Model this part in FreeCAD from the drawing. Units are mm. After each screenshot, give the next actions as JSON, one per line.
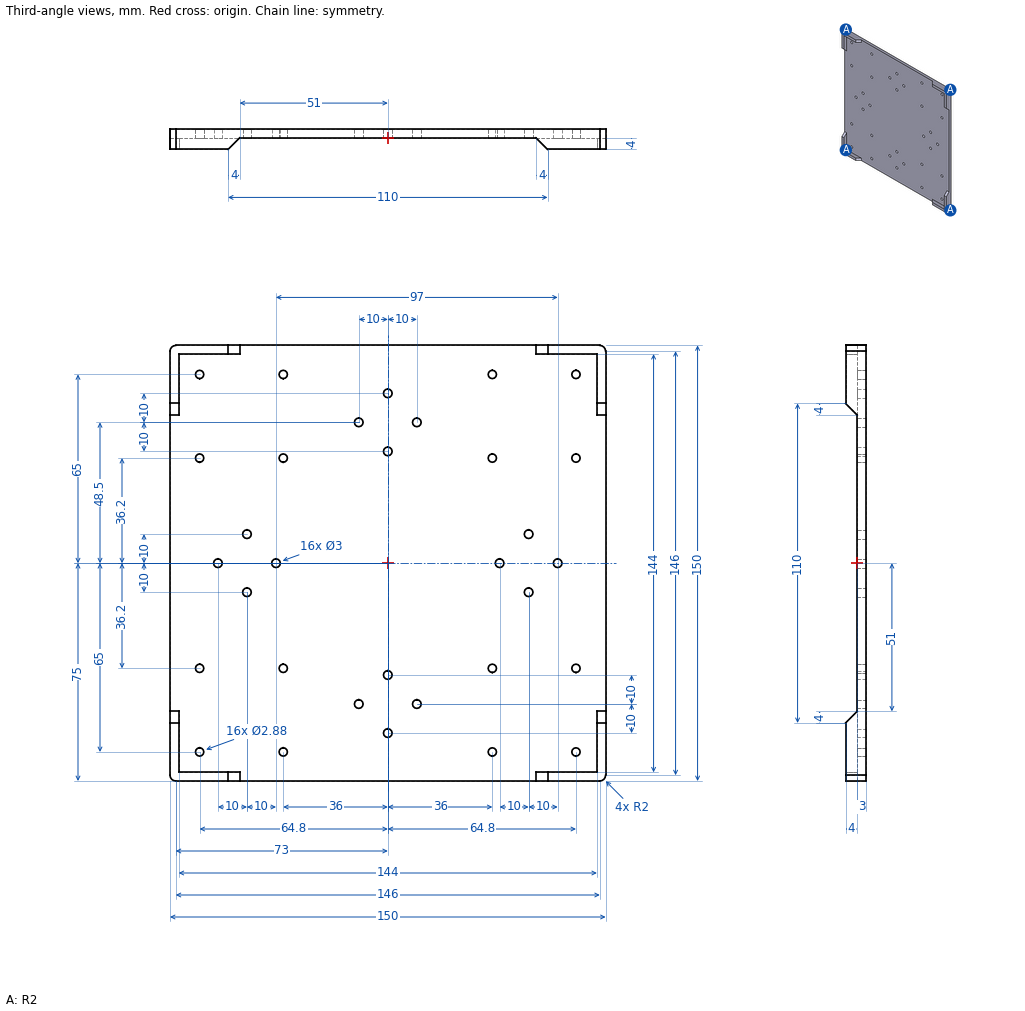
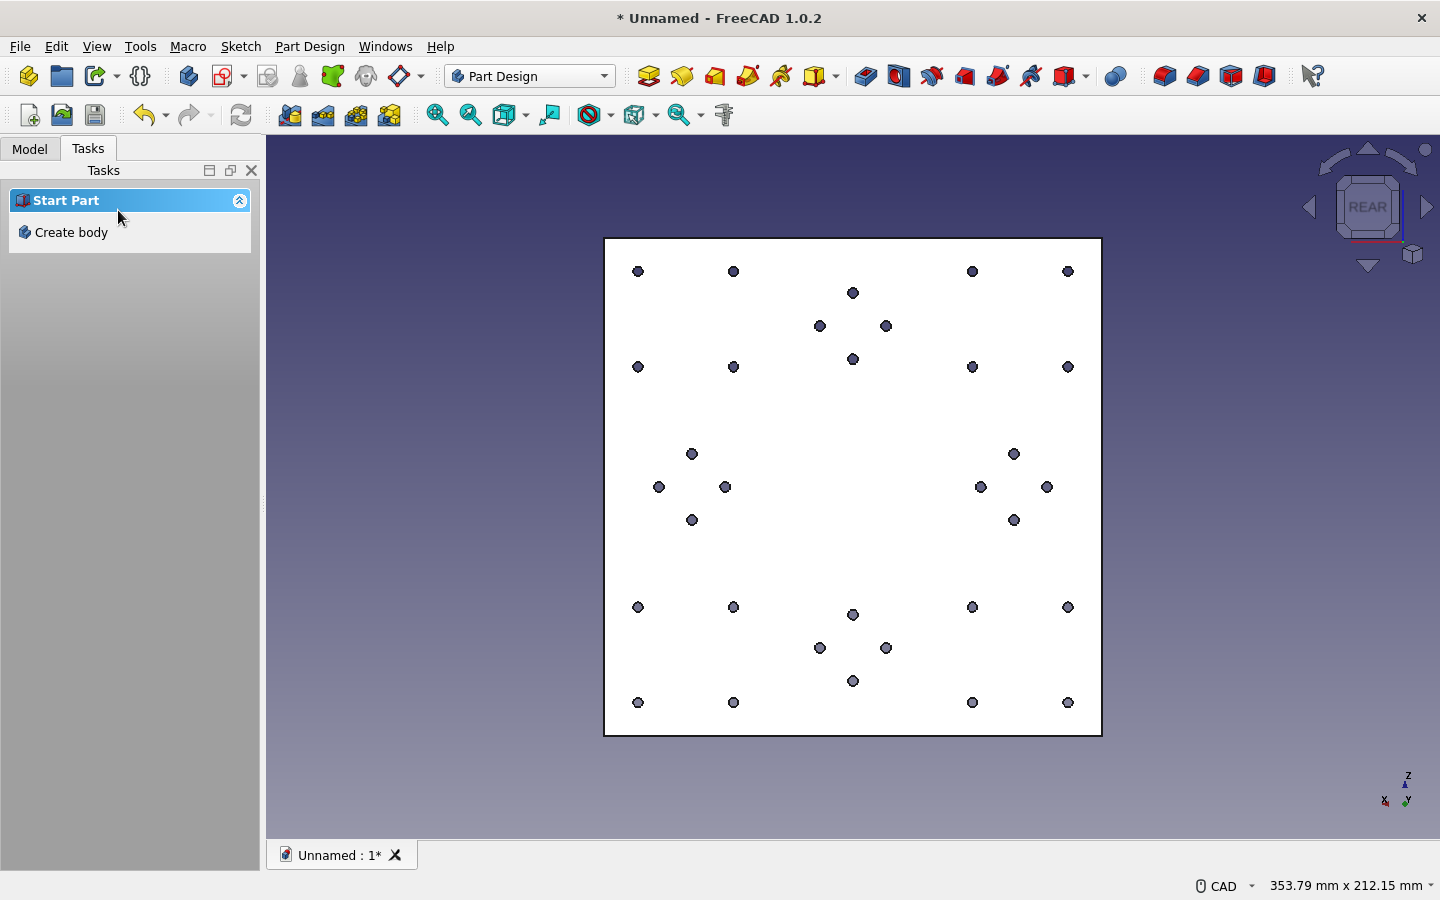
{"action": "scroll", "coordinate": [604, 237], "scroll_direction": "up", "scroll_amount": 7}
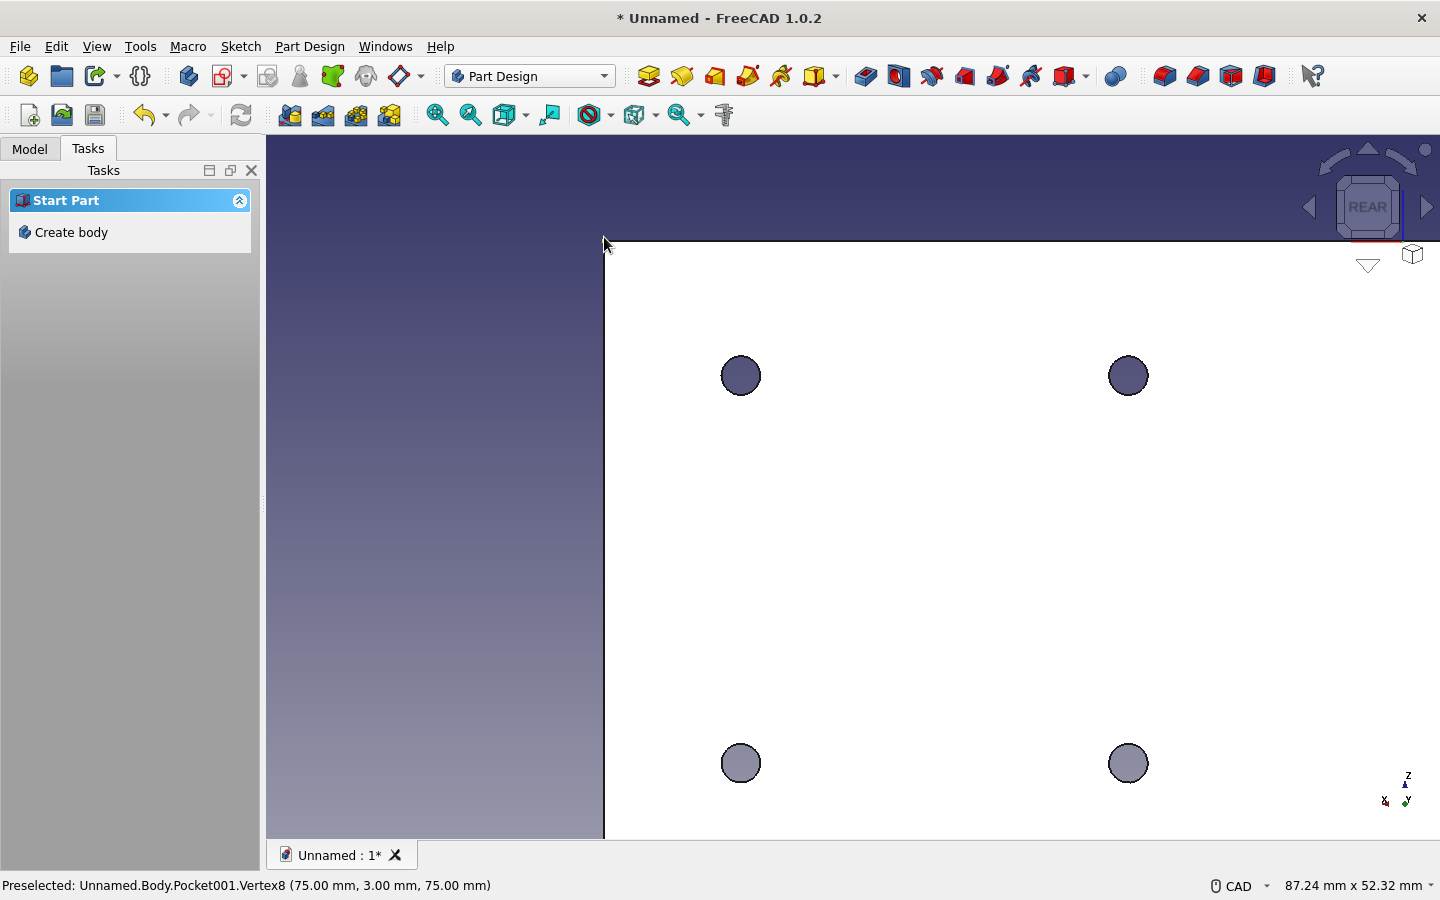
{"action": "key", "text": "v f"}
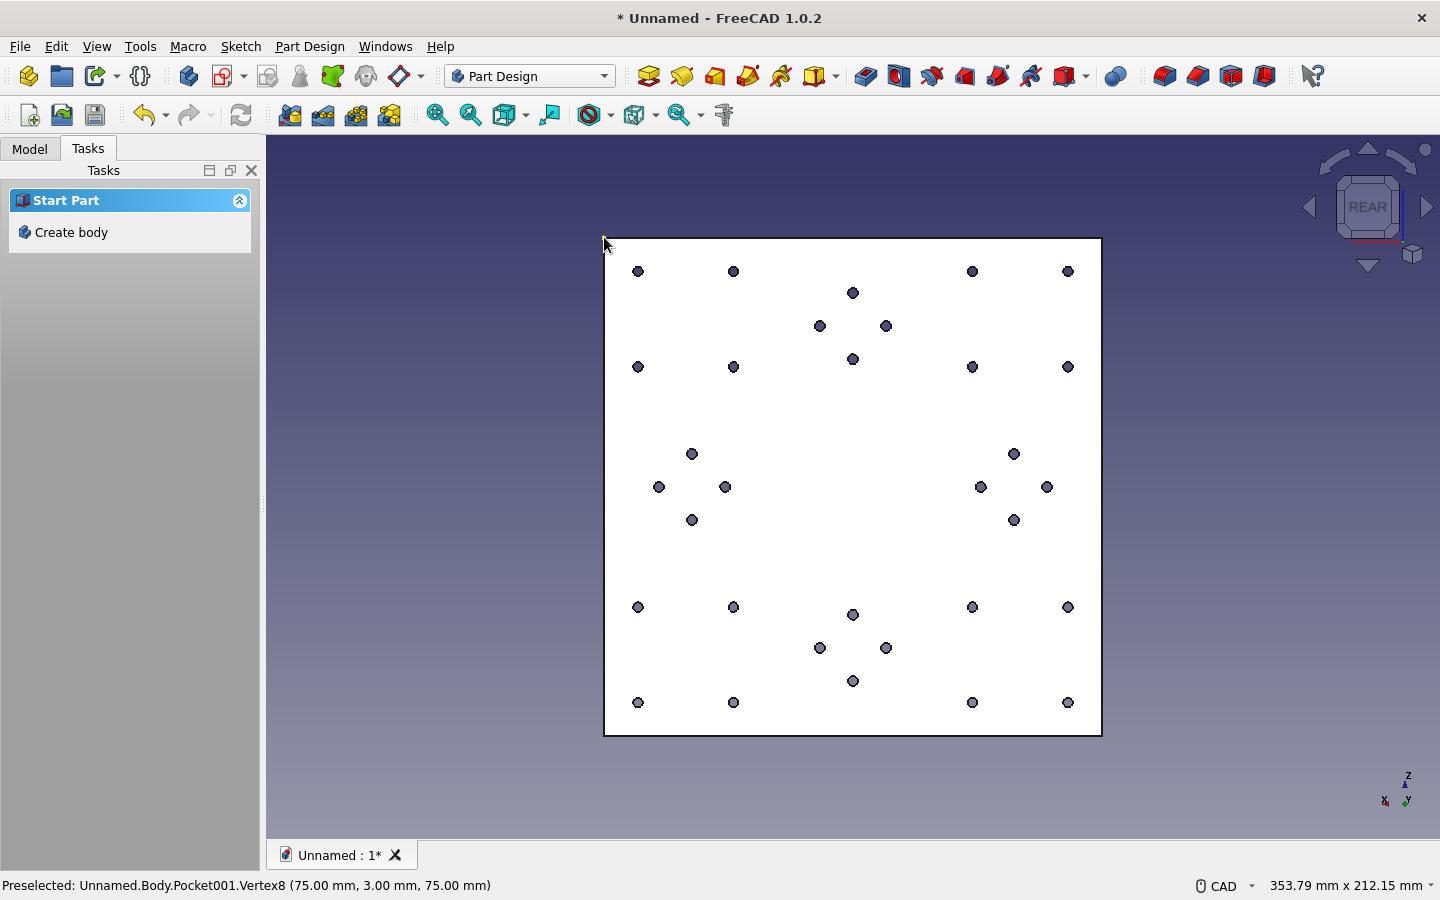
{"action": "key", "text": "0"}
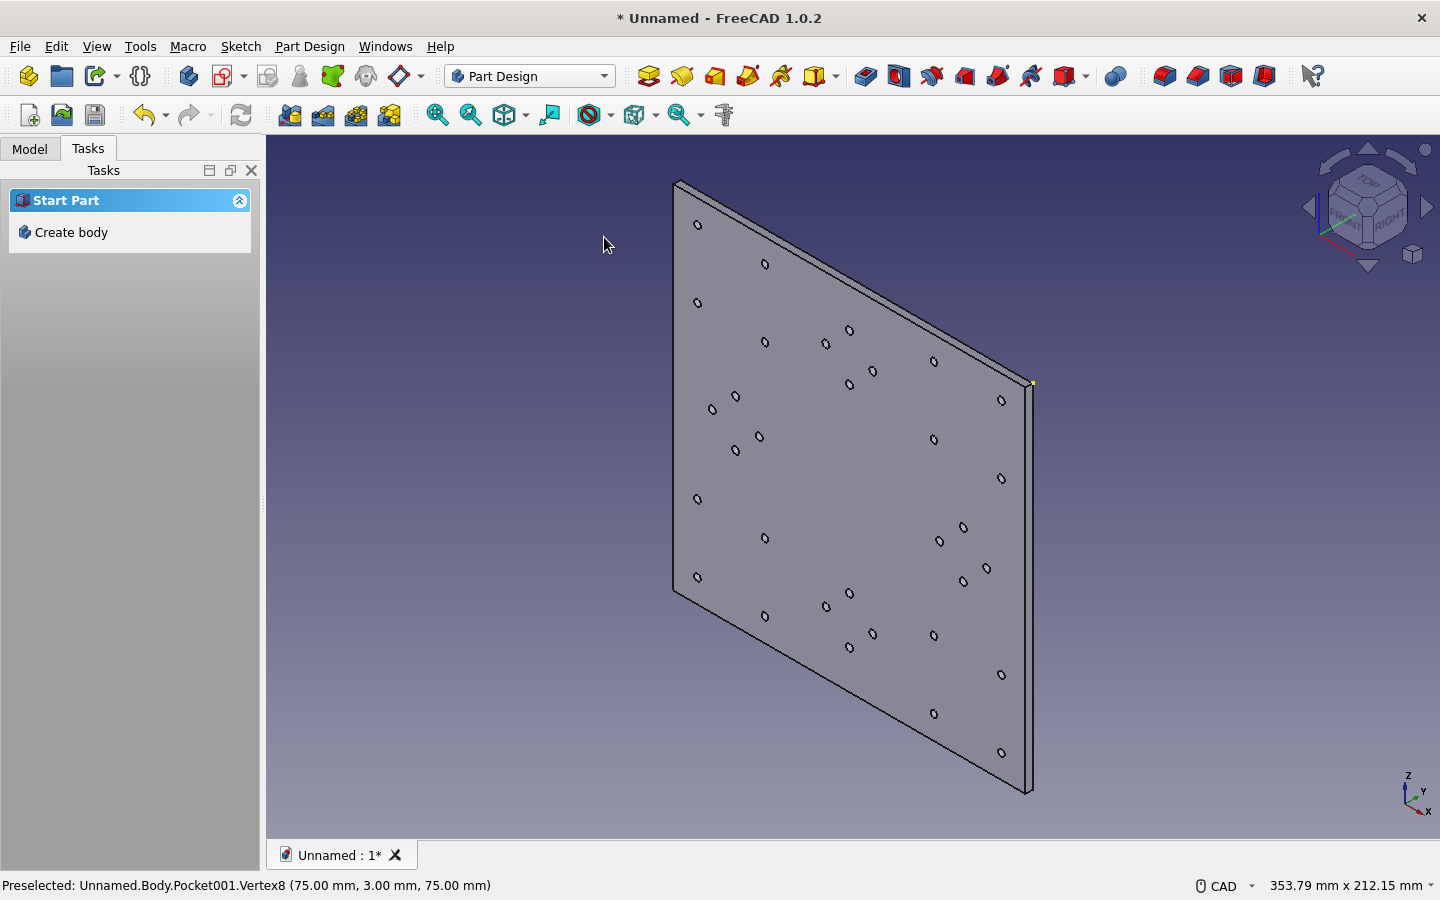
{"action": "left_click", "coordinate": [1031, 383]}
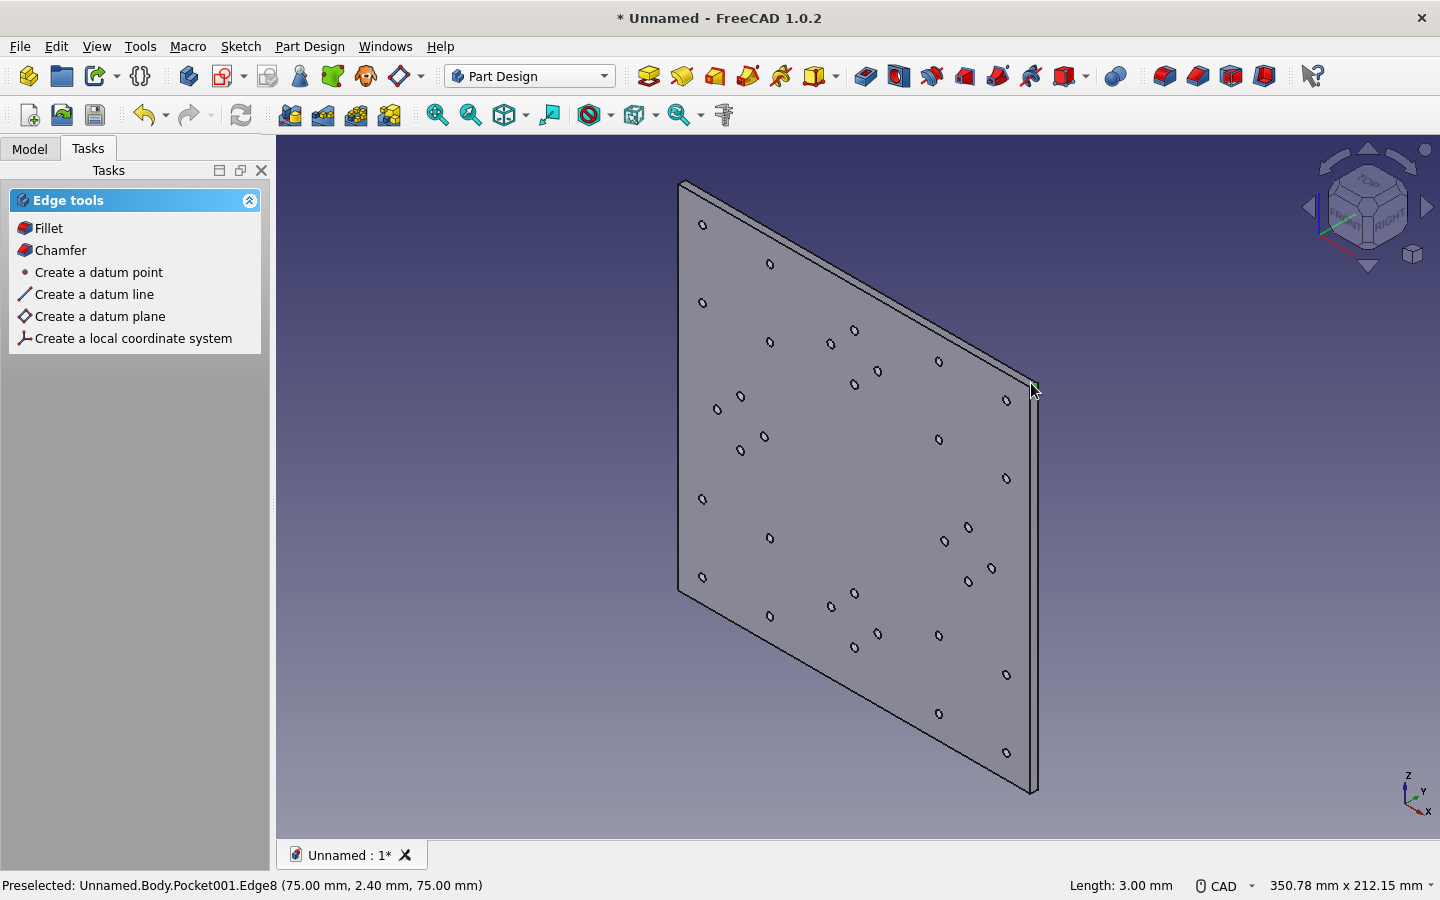
{"action": "scroll", "coordinate": [682, 181], "scroll_direction": "up", "scroll_amount": 7}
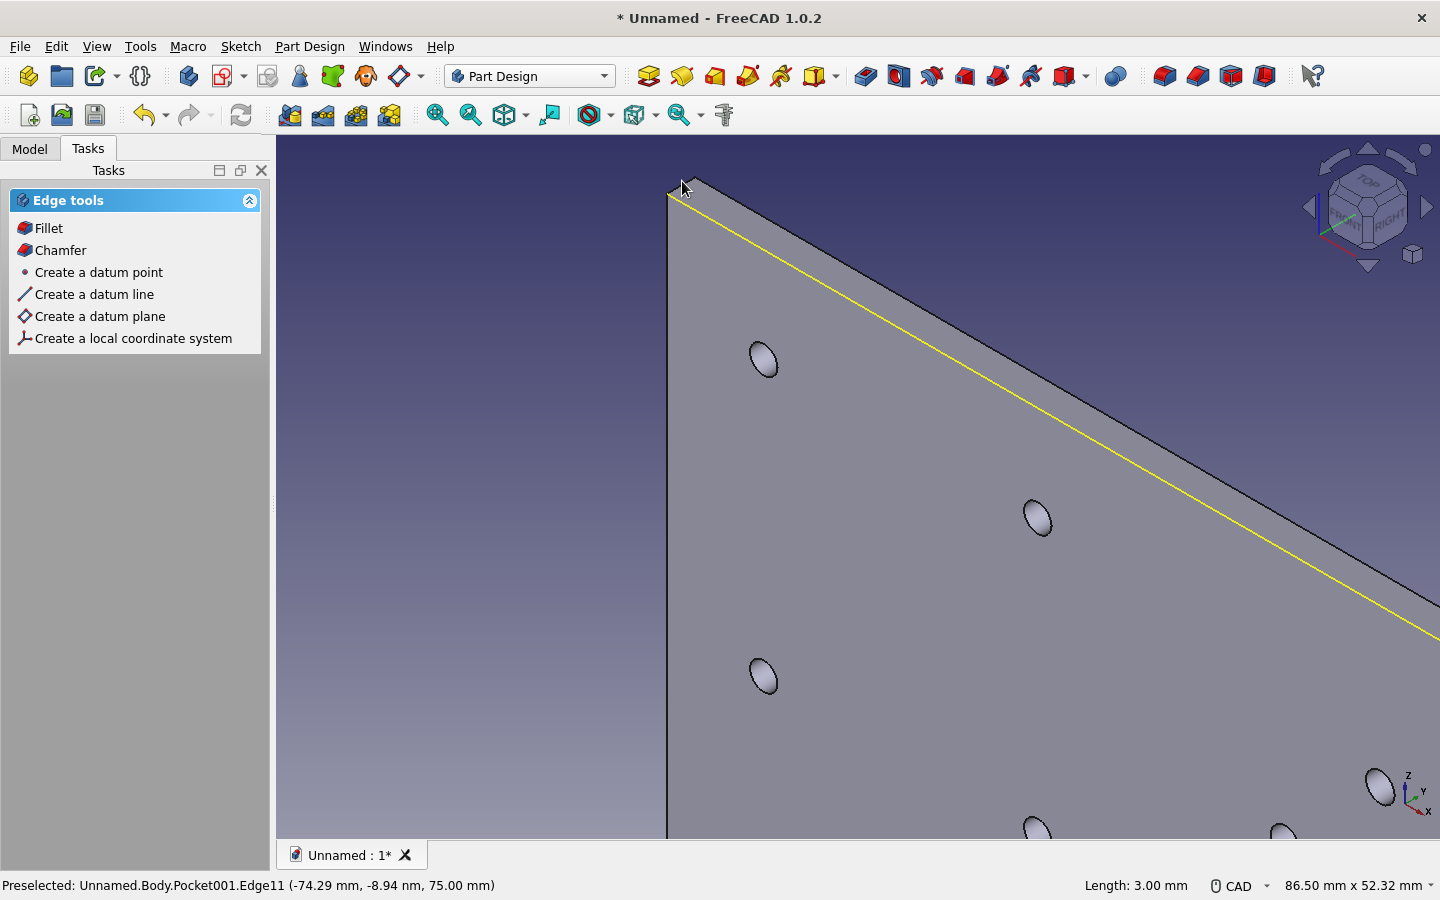
{"action": "key", "text": "v f"}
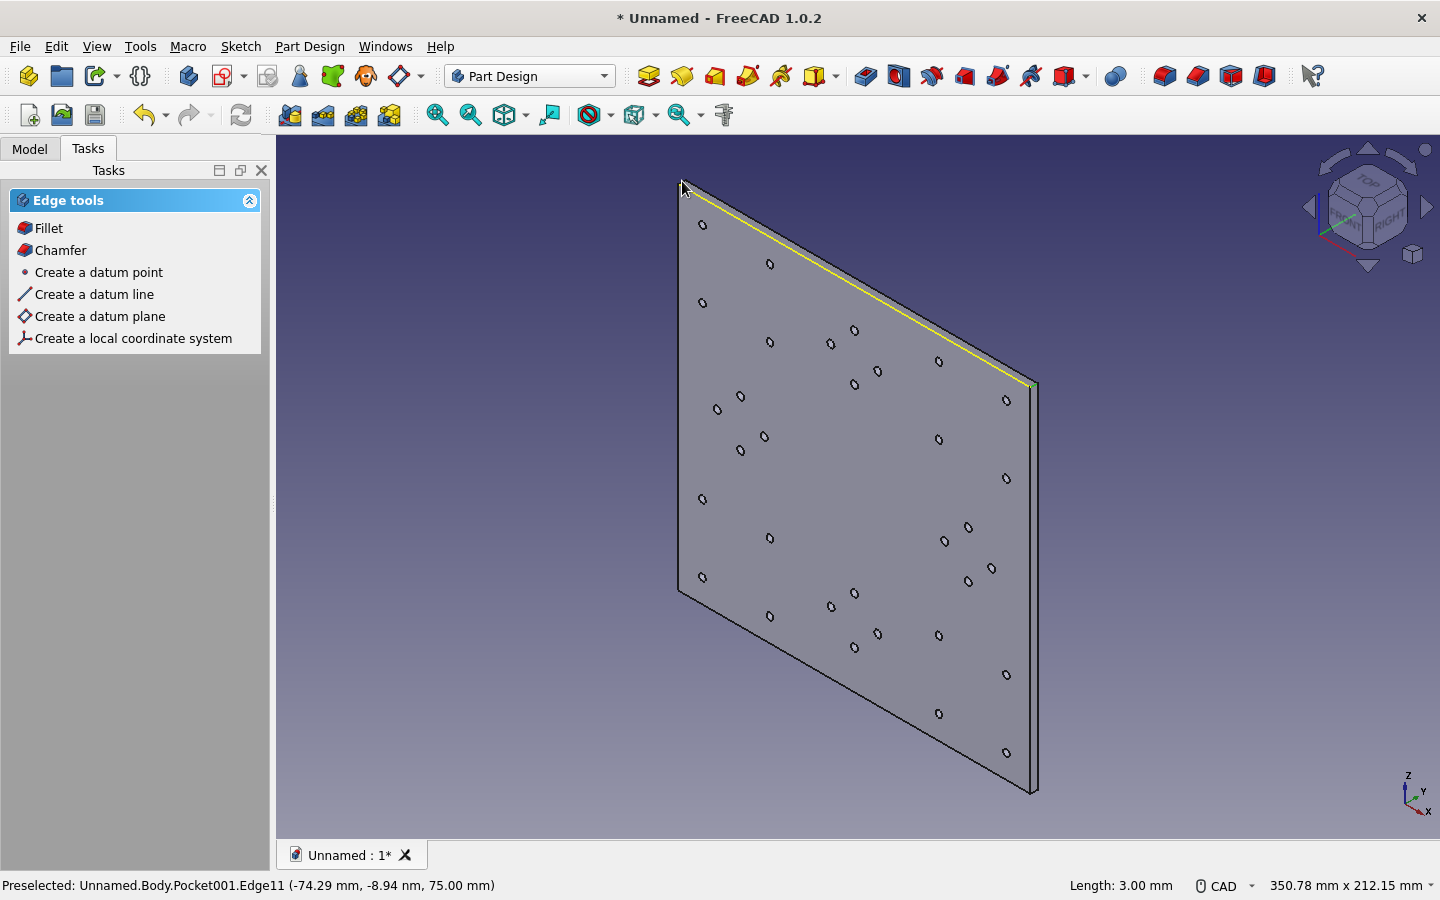
{"action": "key", "text": "2"}